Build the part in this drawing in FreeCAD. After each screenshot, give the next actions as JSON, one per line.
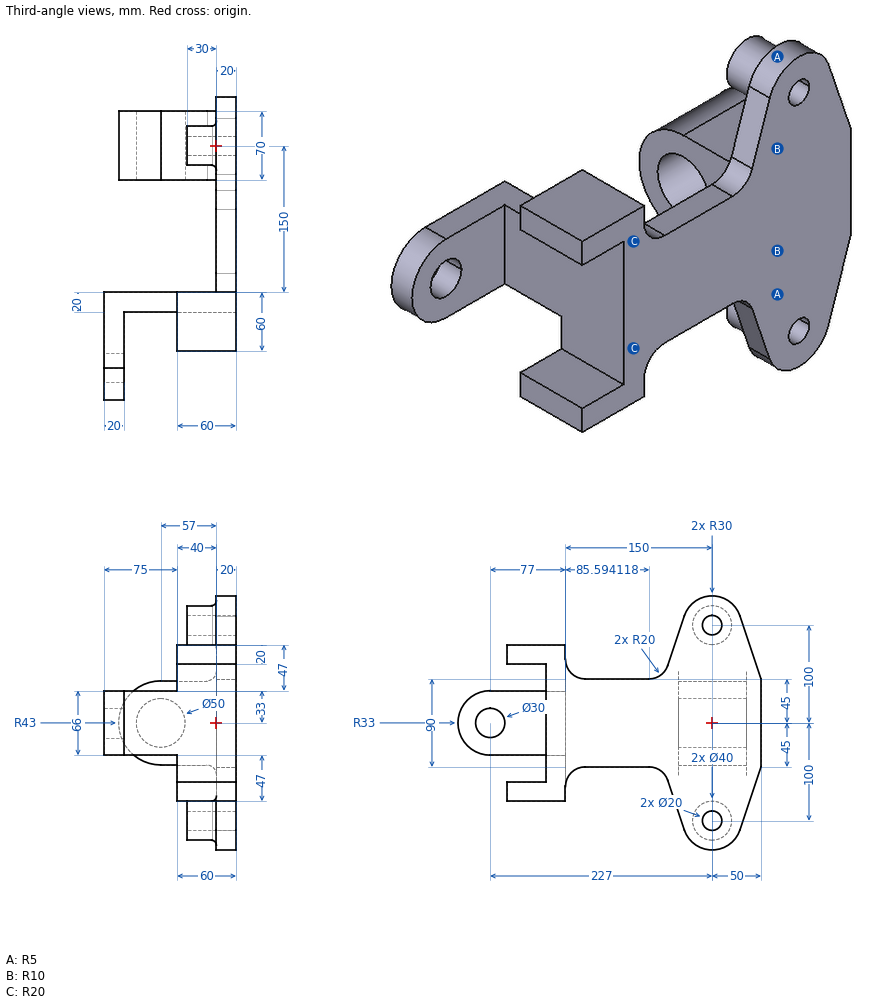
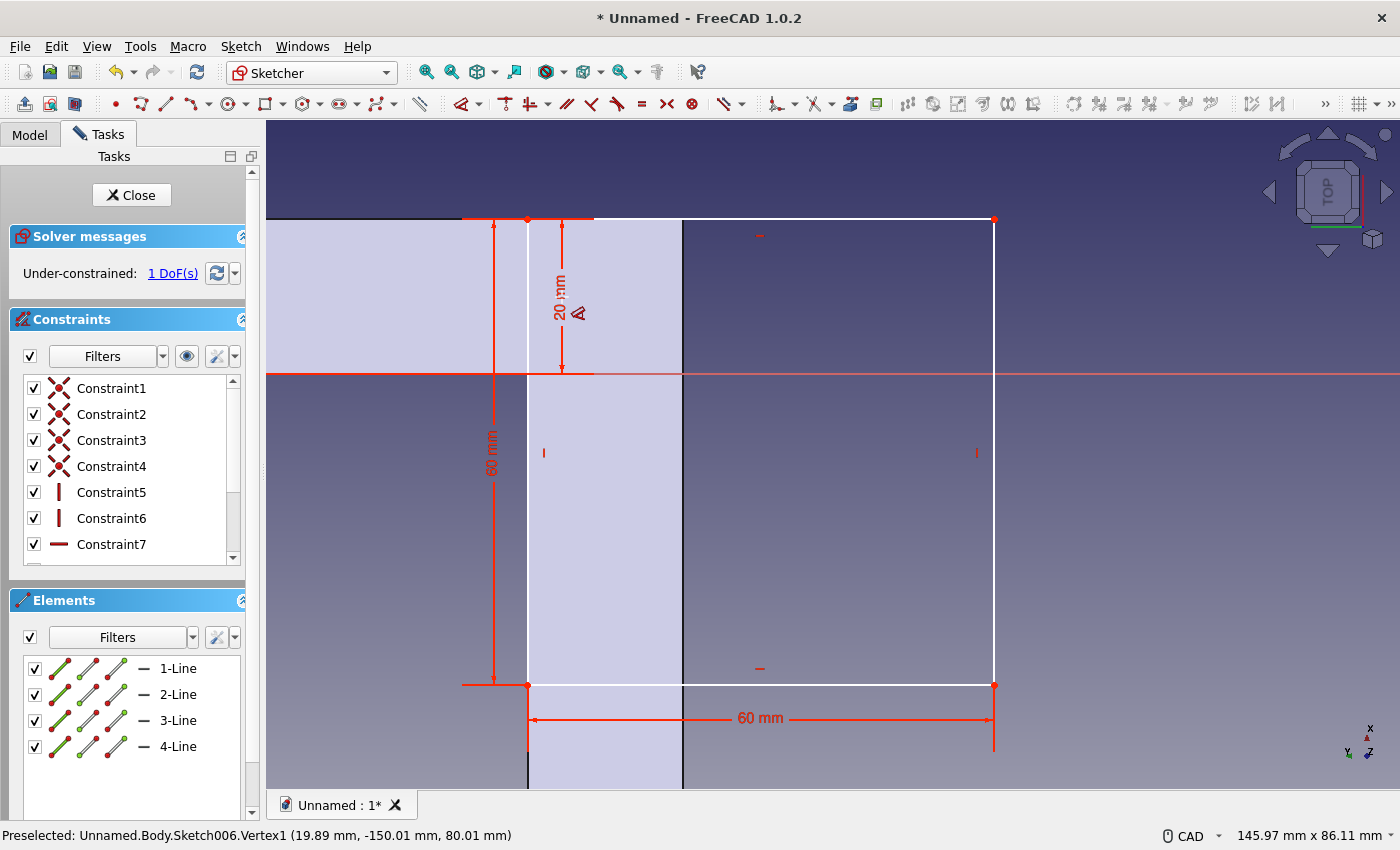
{"action": "left_click", "coordinate": [528, 219]}
{"action": "left_click", "coordinate": [411, 185]}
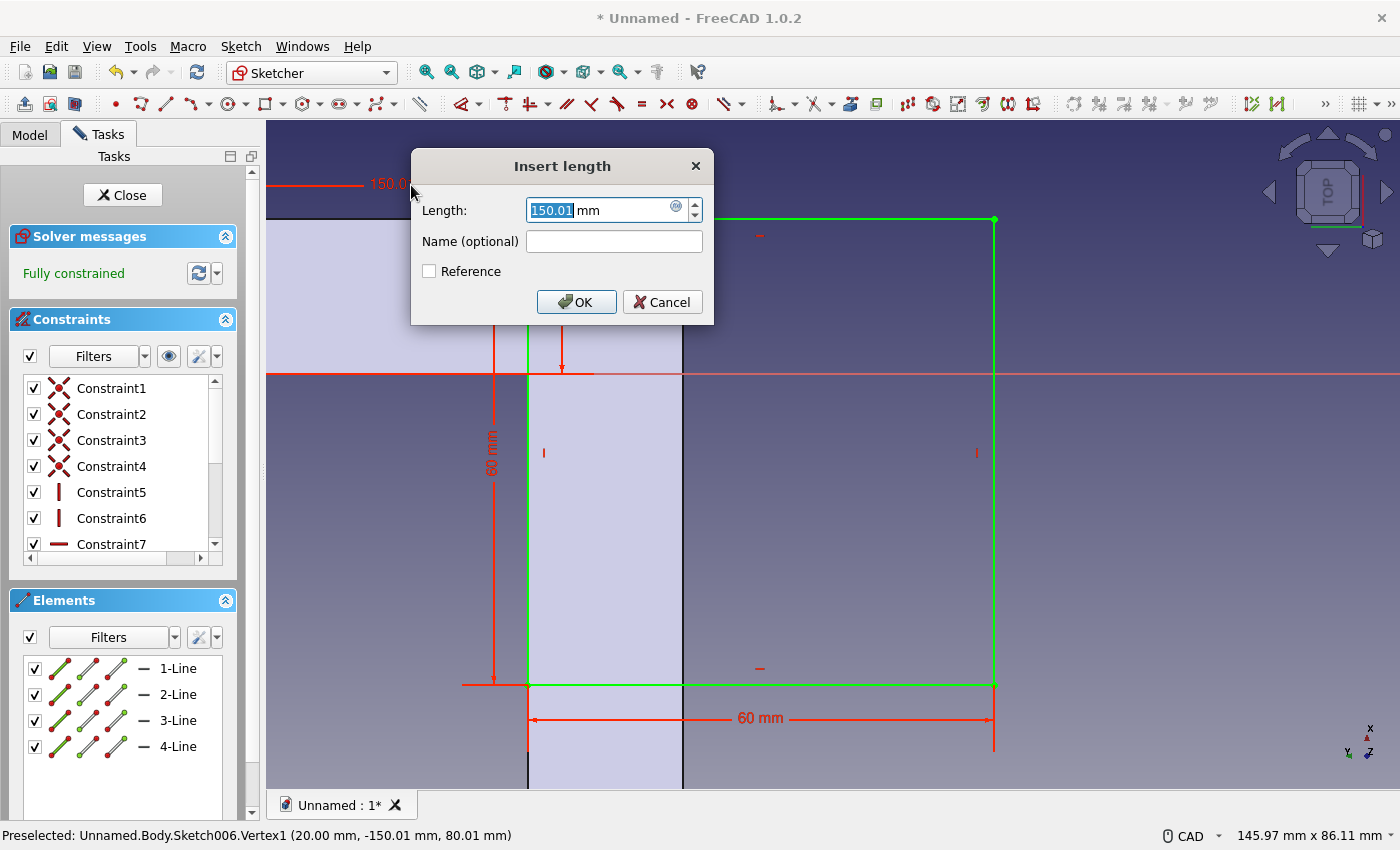
{"action": "type", "text": "150"}
{"action": "key", "text": "Return"}
{"action": "key", "text": "Escape"}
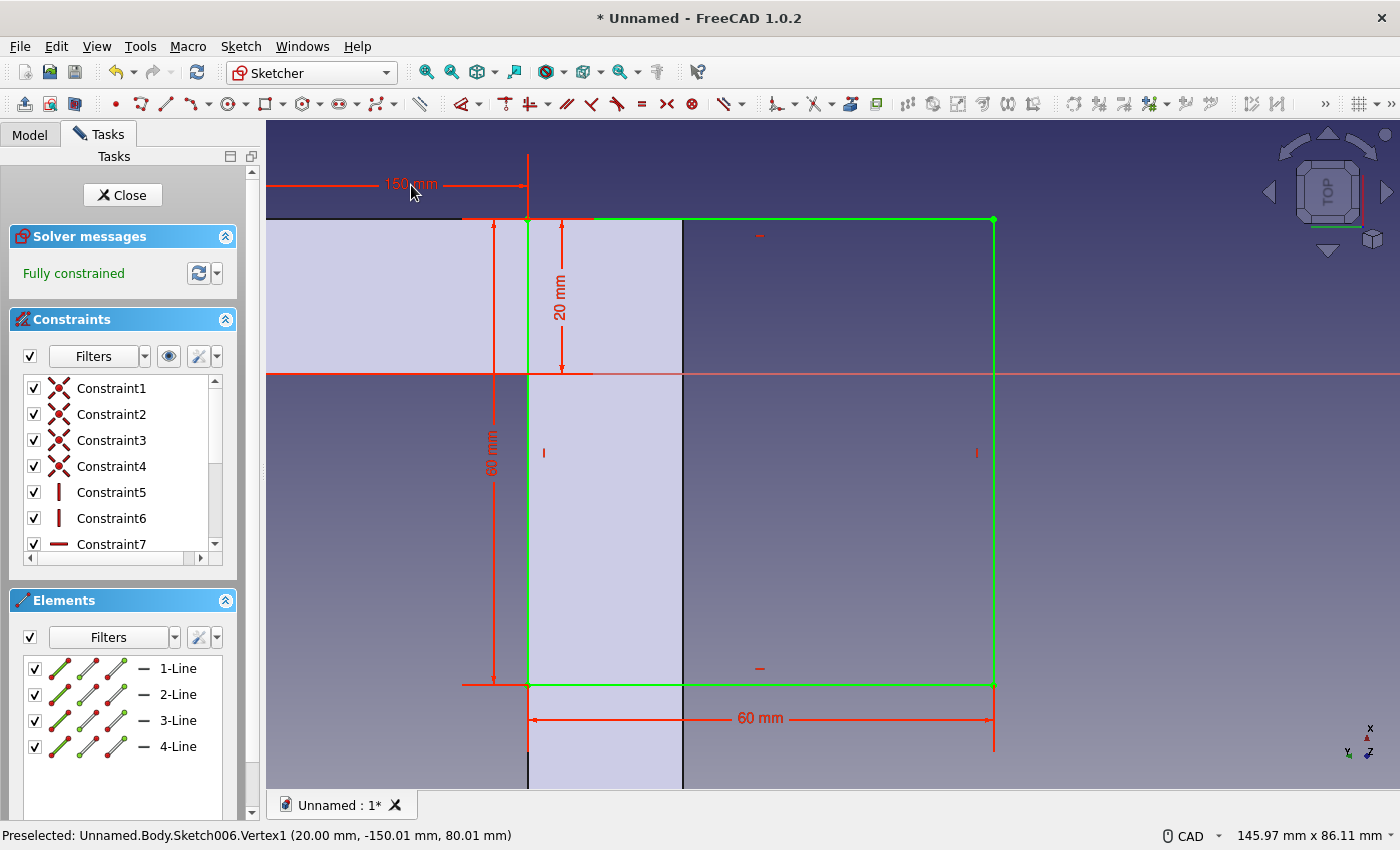
{"action": "left_click", "coordinate": [123, 195]}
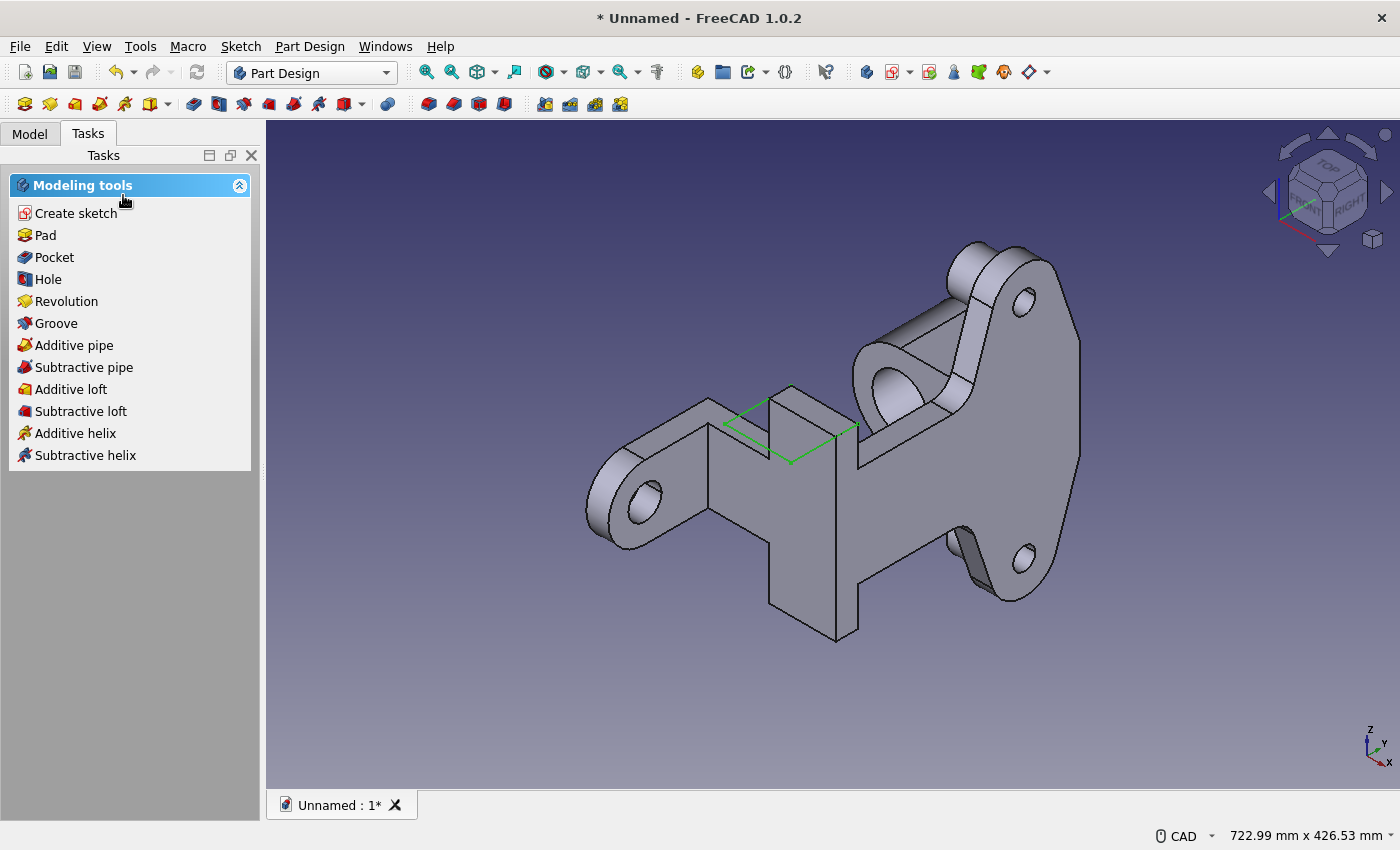
{"action": "left_click", "coordinate": [25, 104]}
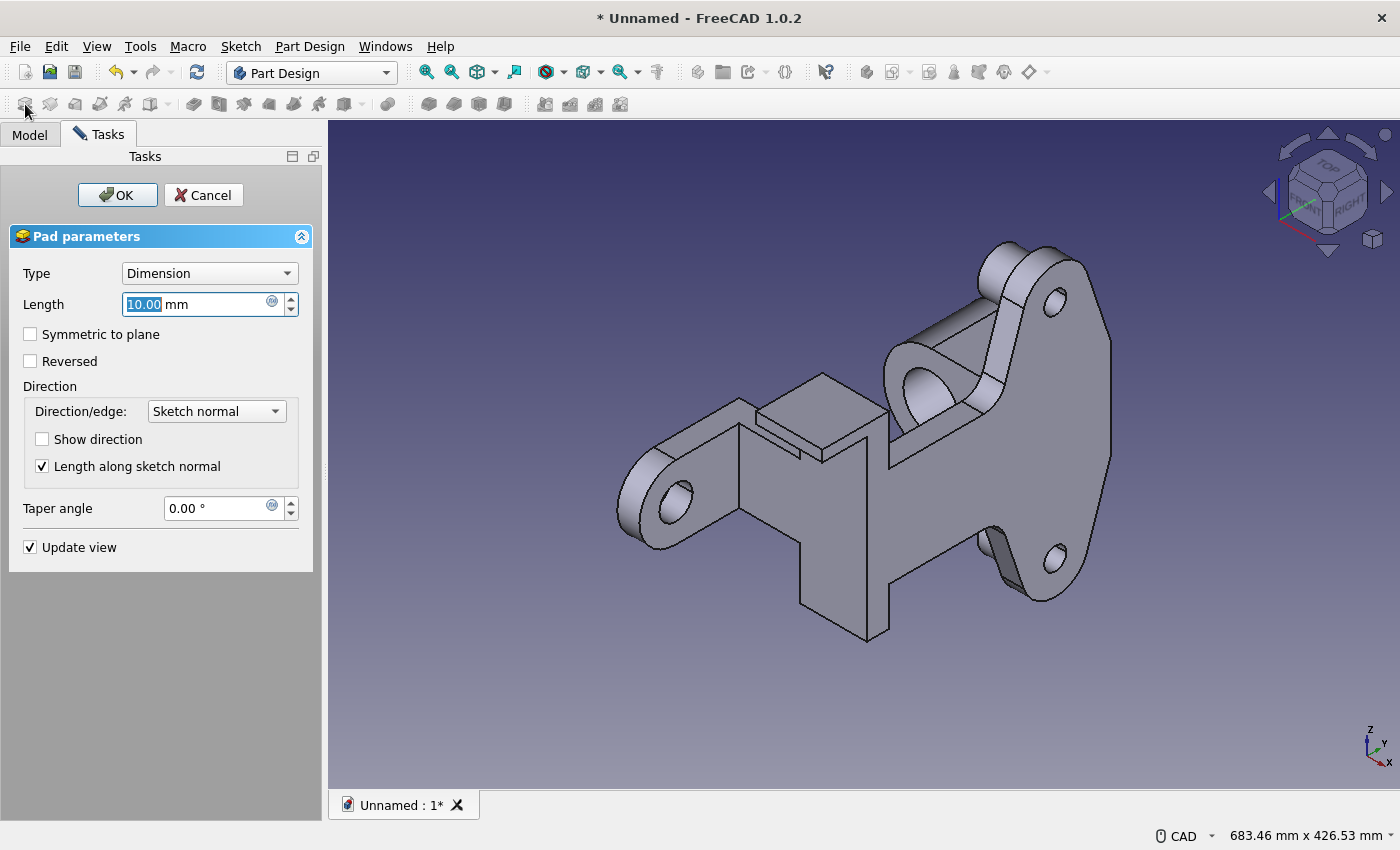
{"action": "type", "text": "20"}
{"action": "key", "text": "Tab"}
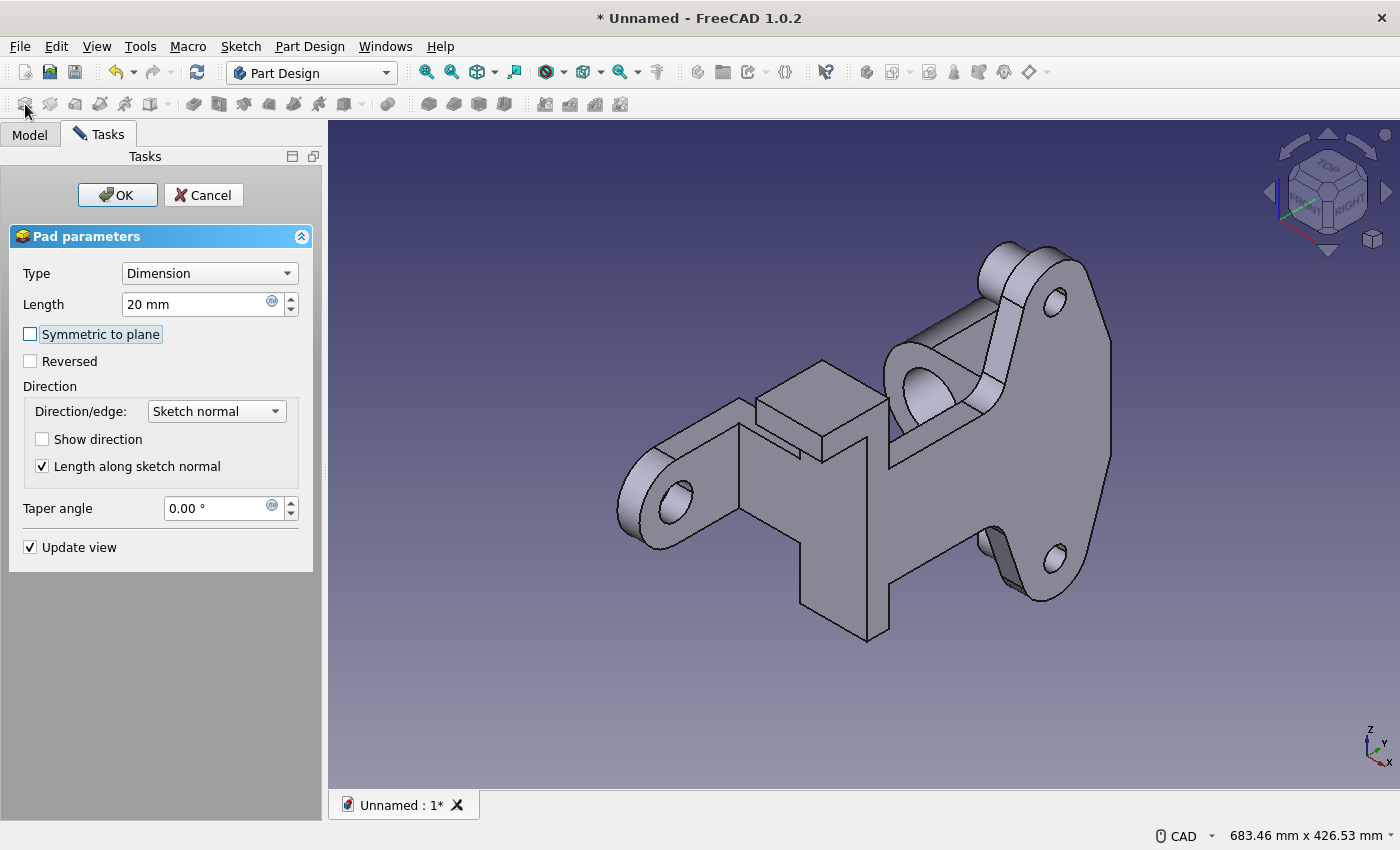
{"action": "left_click", "coordinate": [31, 361]}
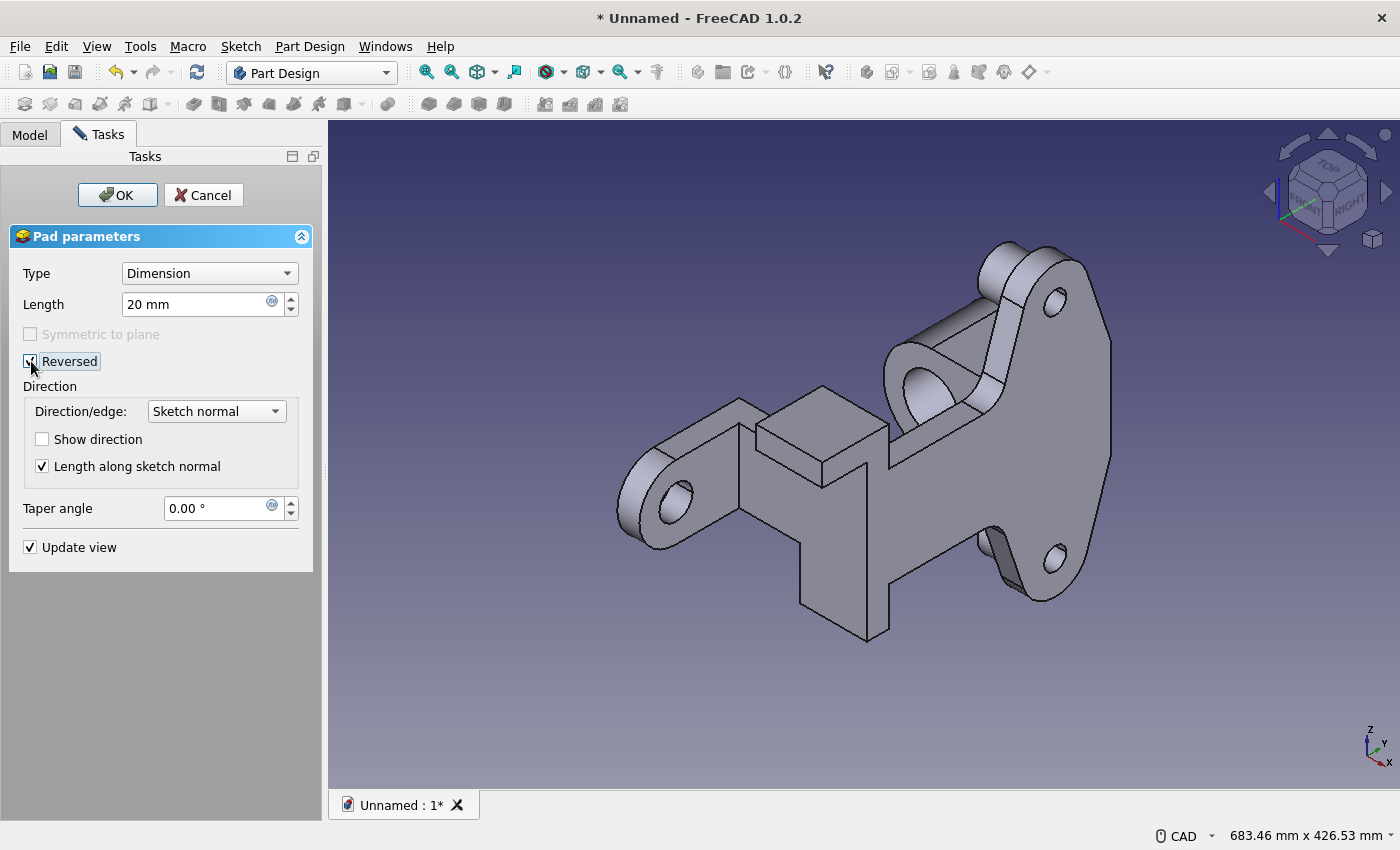
{"action": "left_click", "coordinate": [118, 195]}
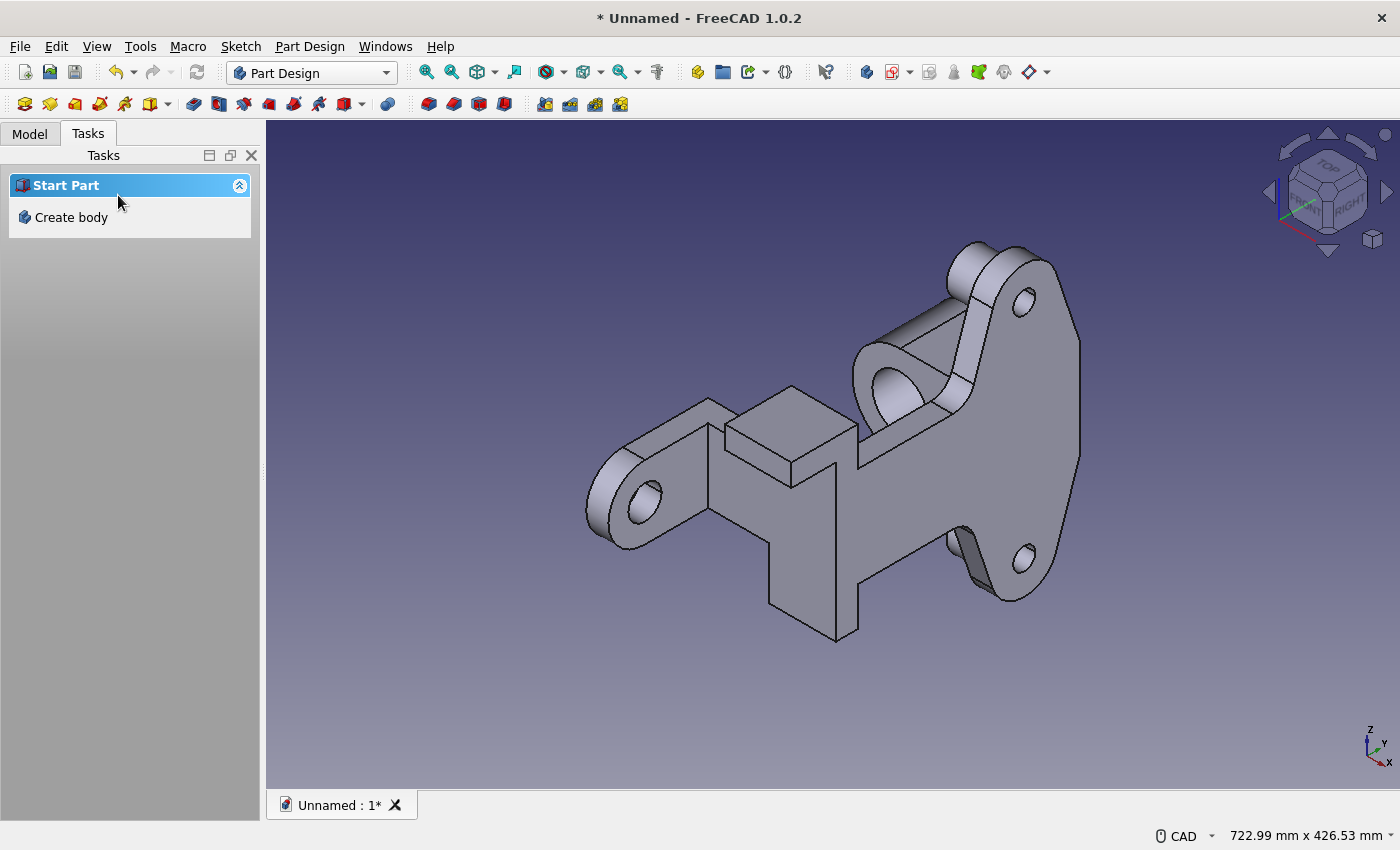
{"action": "left_click", "coordinate": [30, 134]}